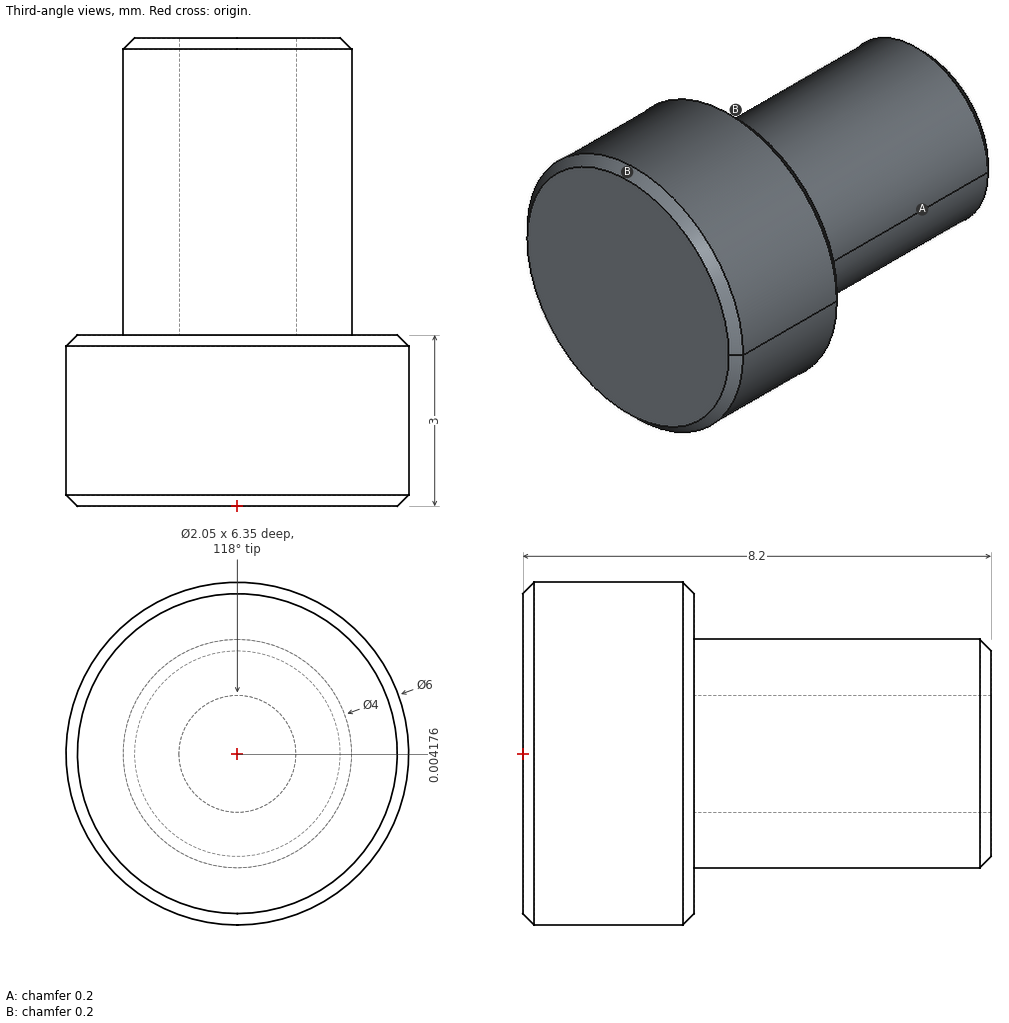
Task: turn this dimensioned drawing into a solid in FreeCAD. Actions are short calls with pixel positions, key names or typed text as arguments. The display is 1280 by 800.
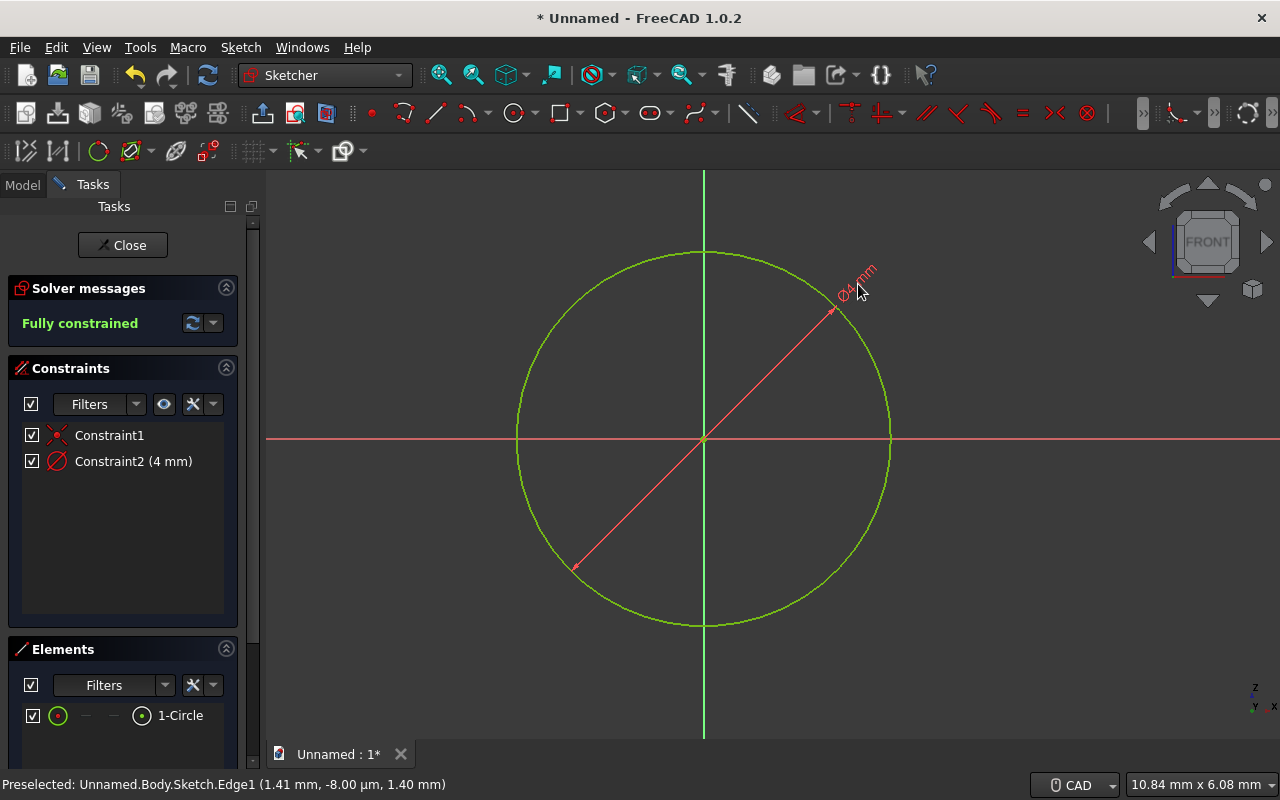
click(123, 245)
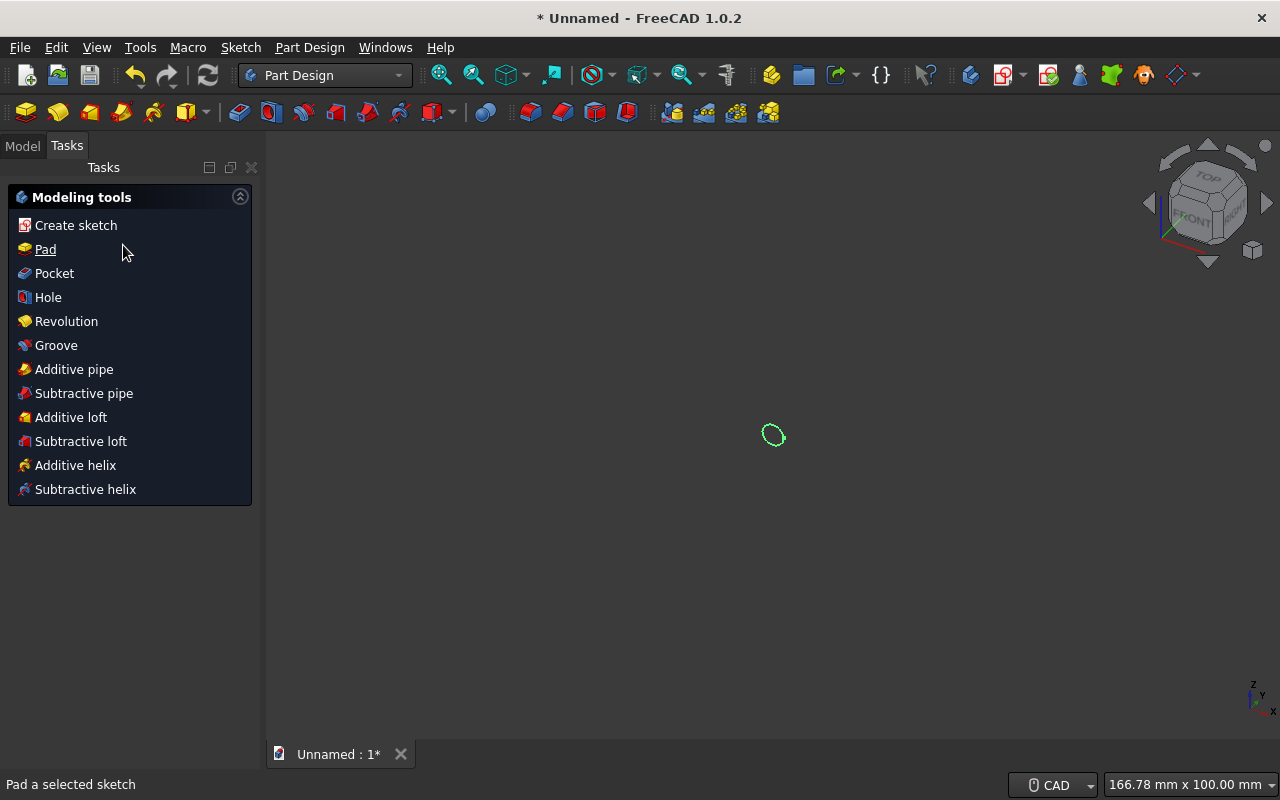
click(26, 112)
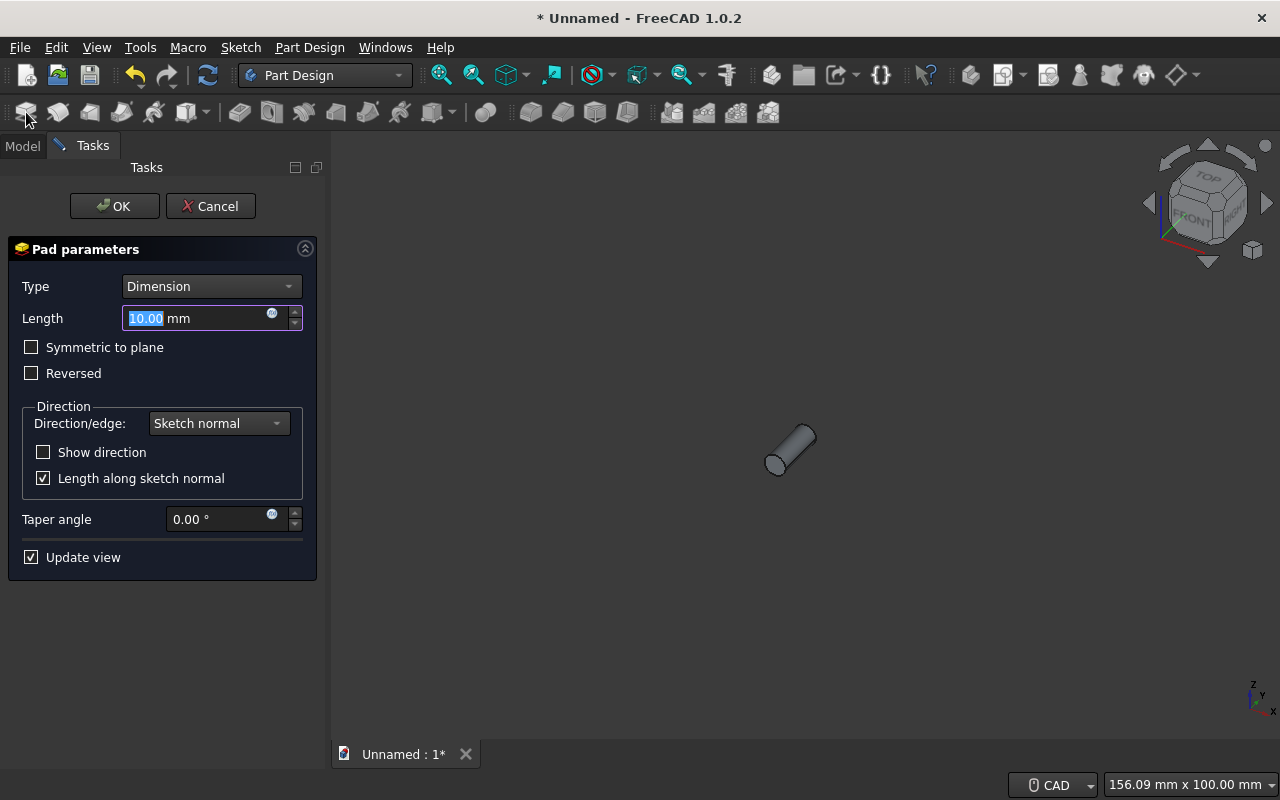
text(8.2)
key(Tab)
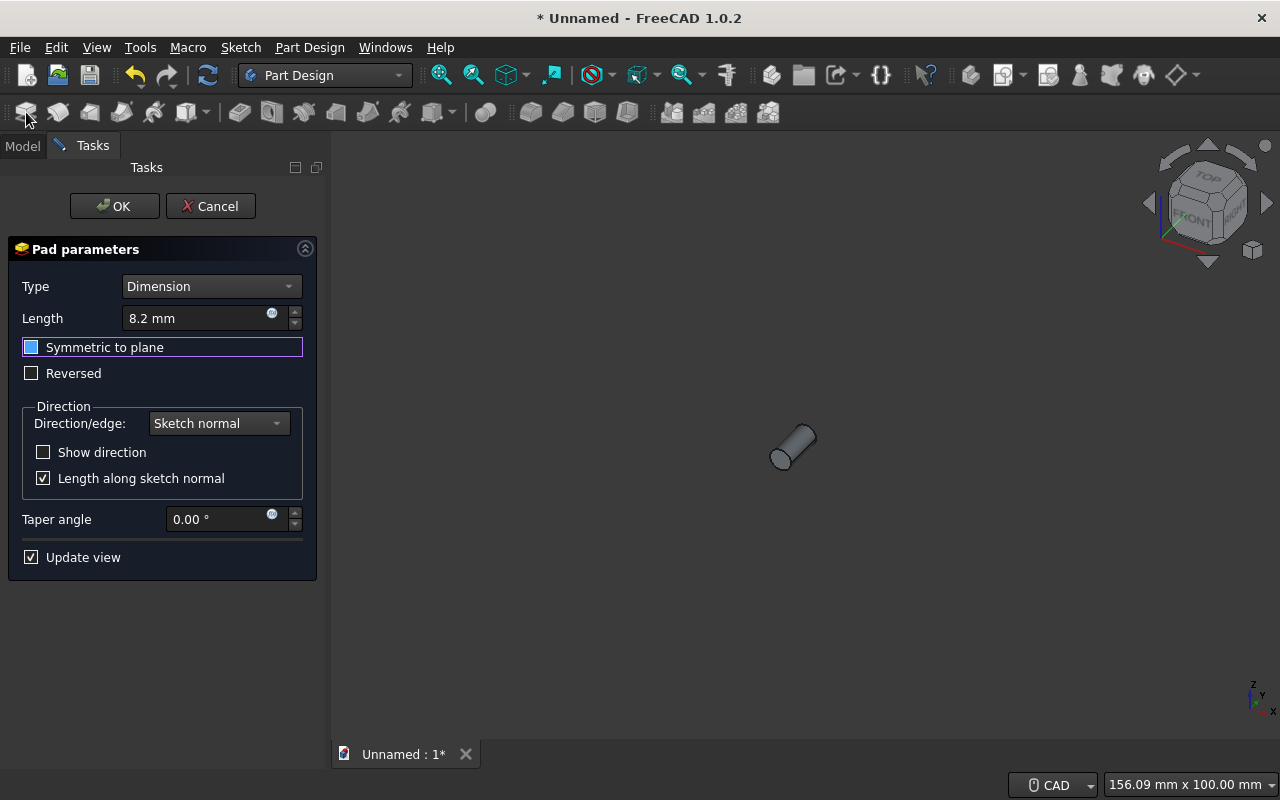
click(30, 373)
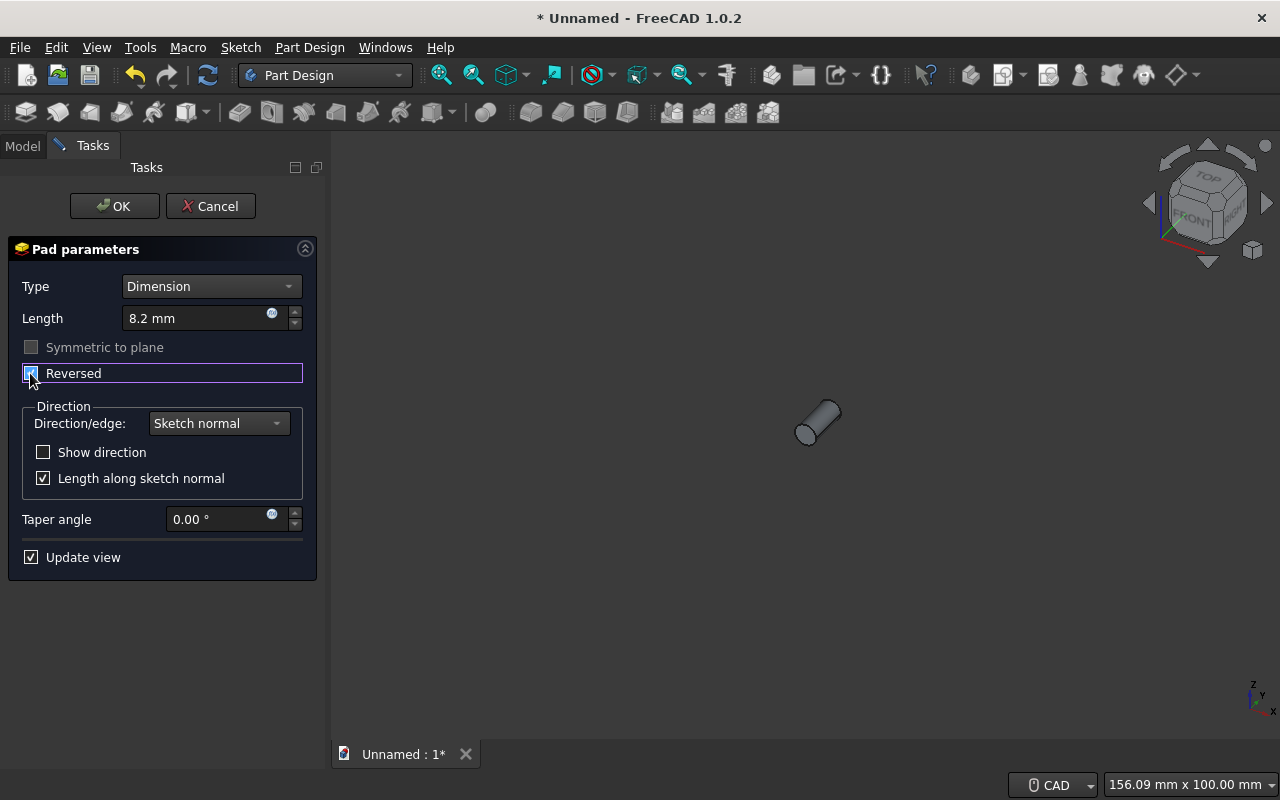
click(115, 206)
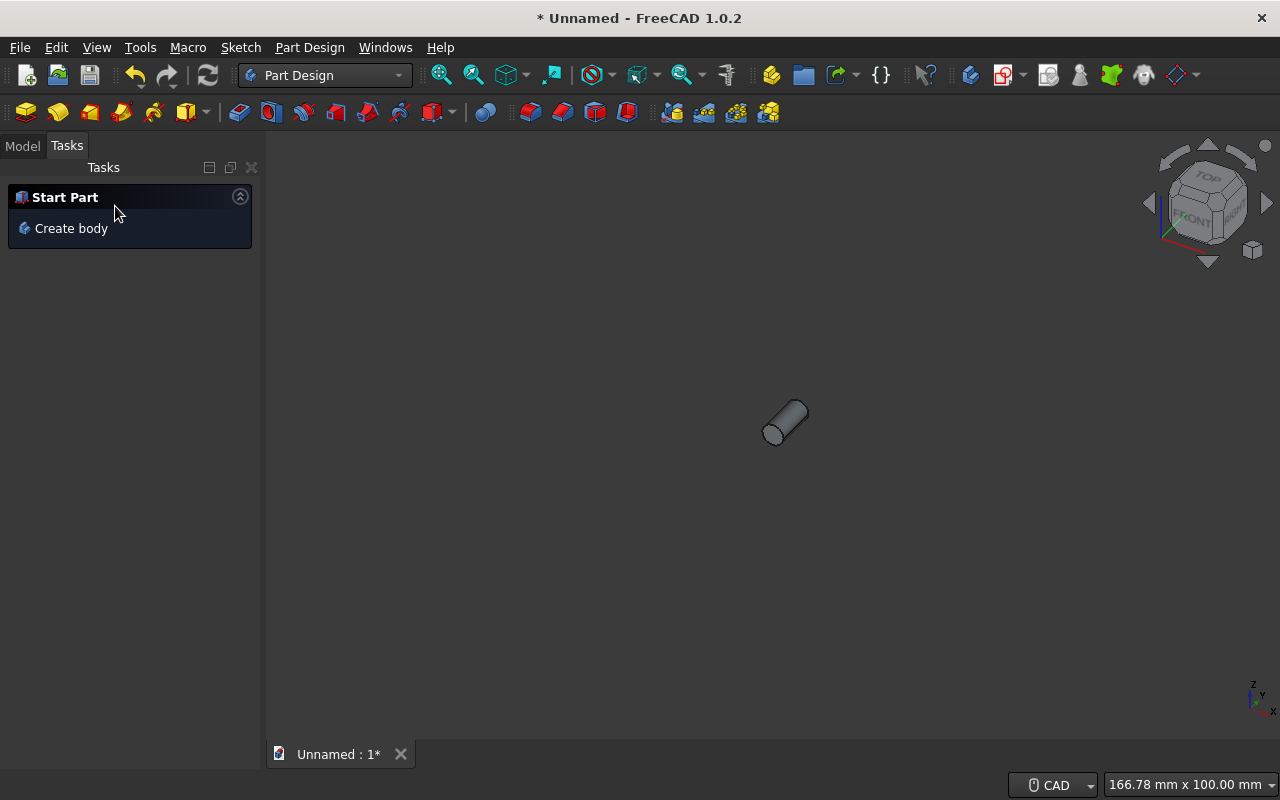
click(442, 76)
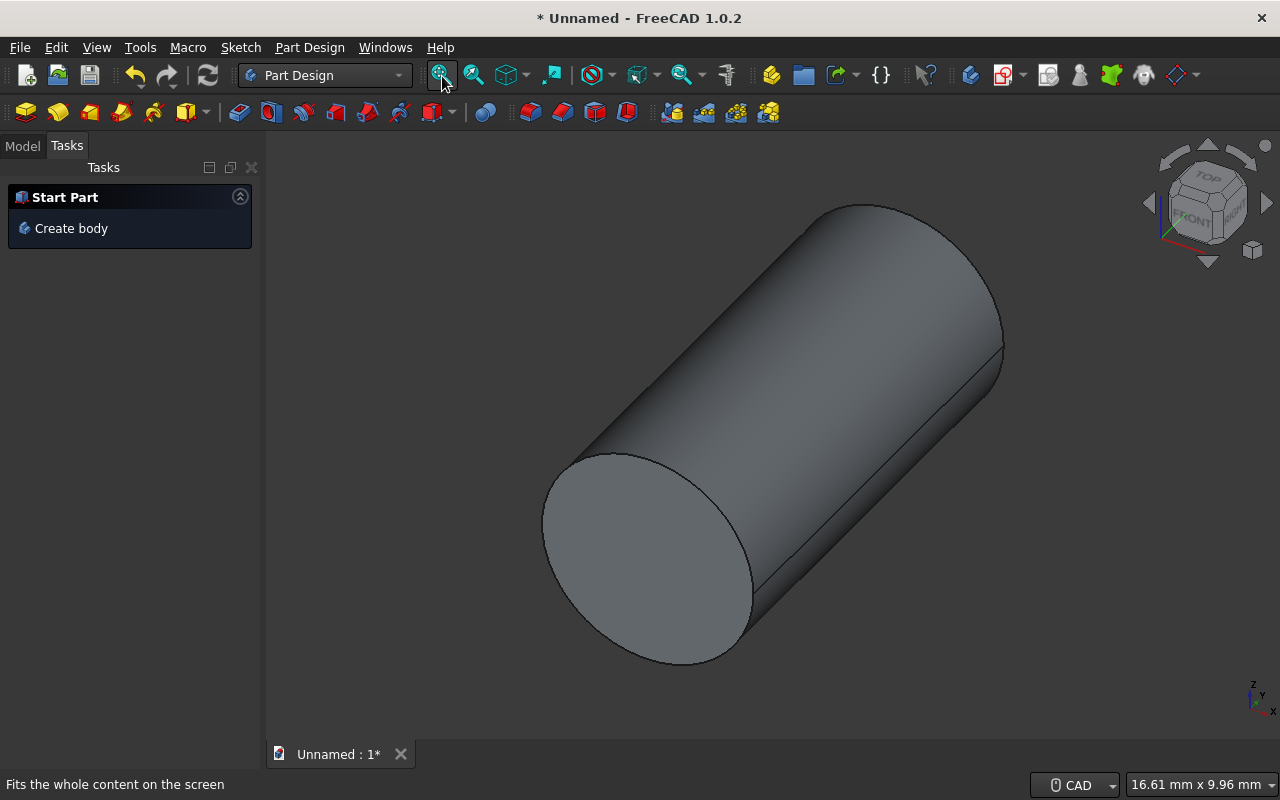
key(4)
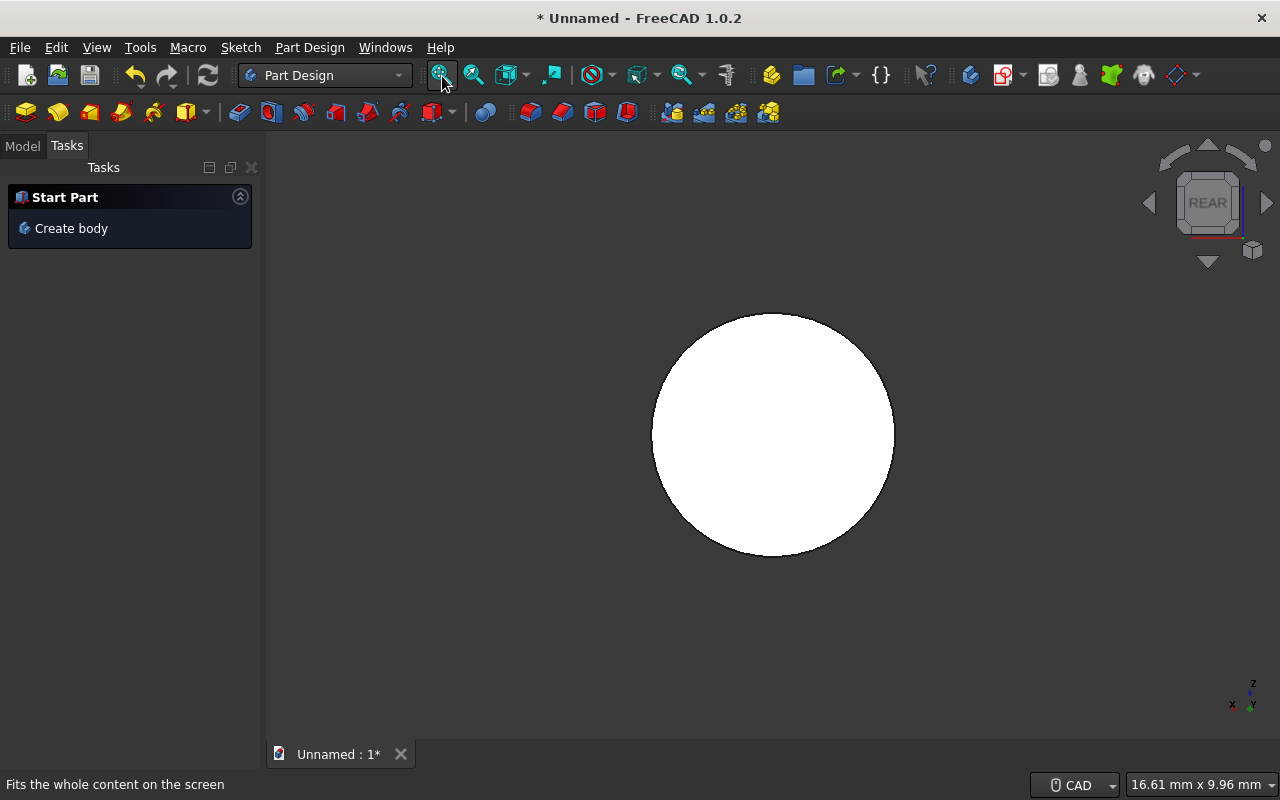
click(442, 76)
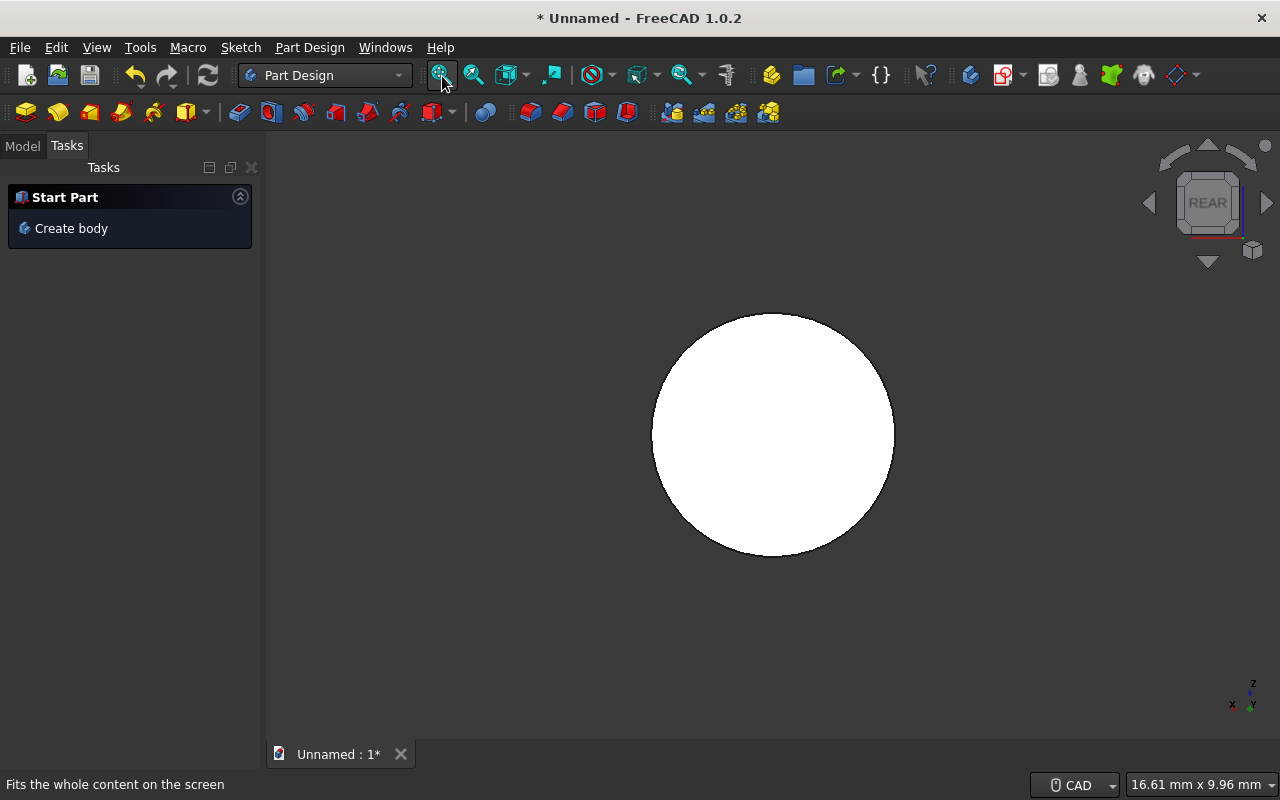
click(773, 434)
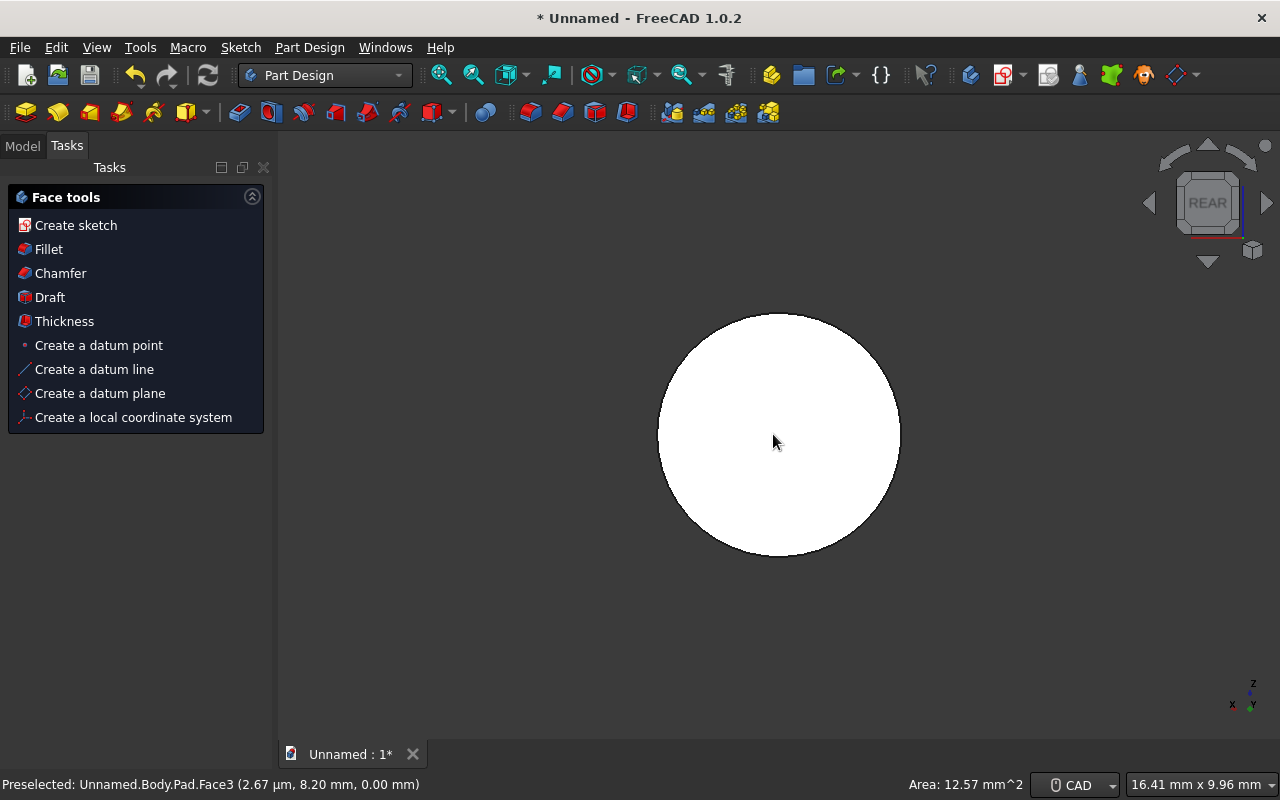
click(1004, 76)